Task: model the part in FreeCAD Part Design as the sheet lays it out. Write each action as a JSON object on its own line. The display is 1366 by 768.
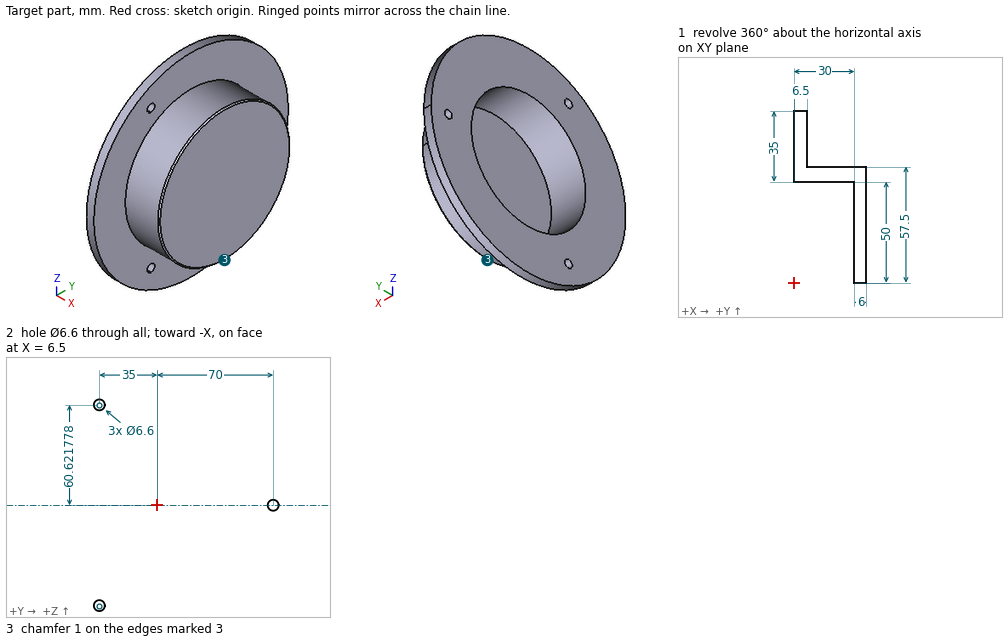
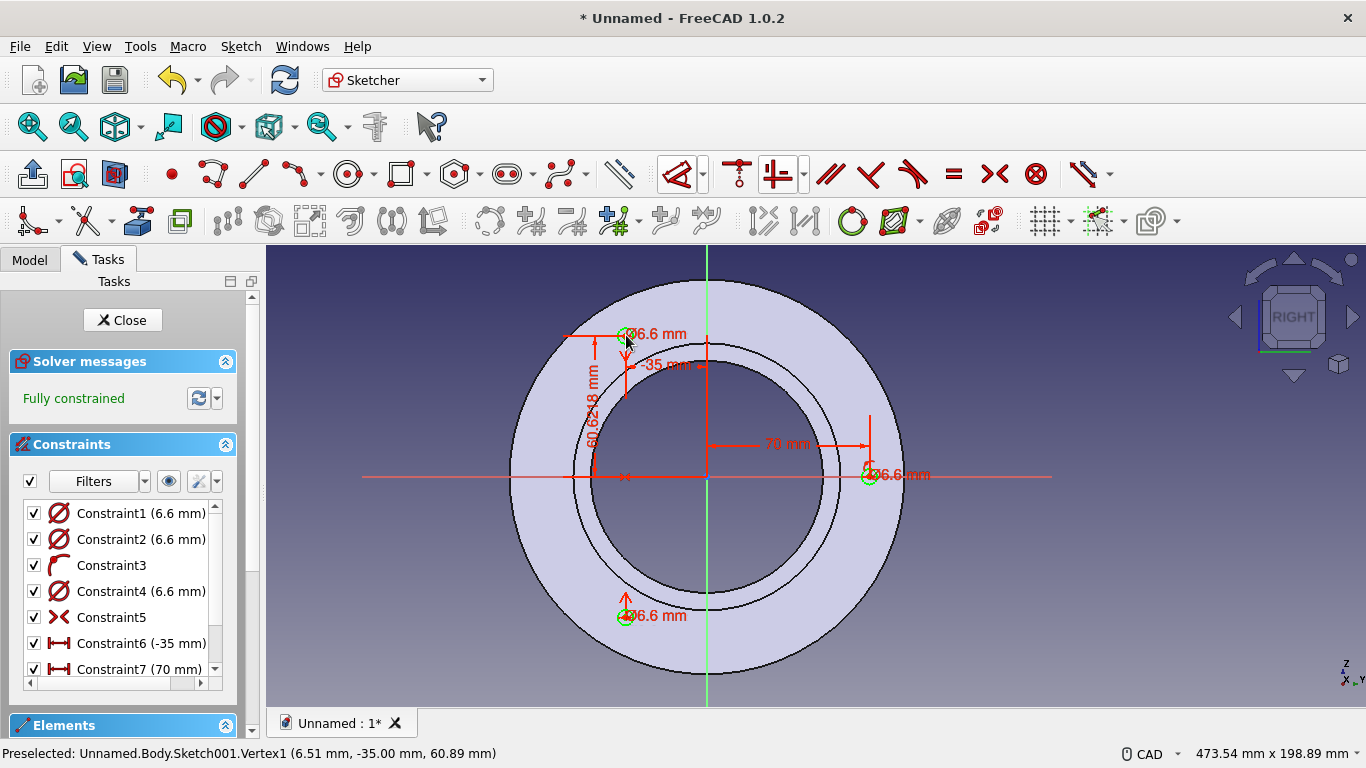
{"action": "left_click", "coordinate": [123, 320]}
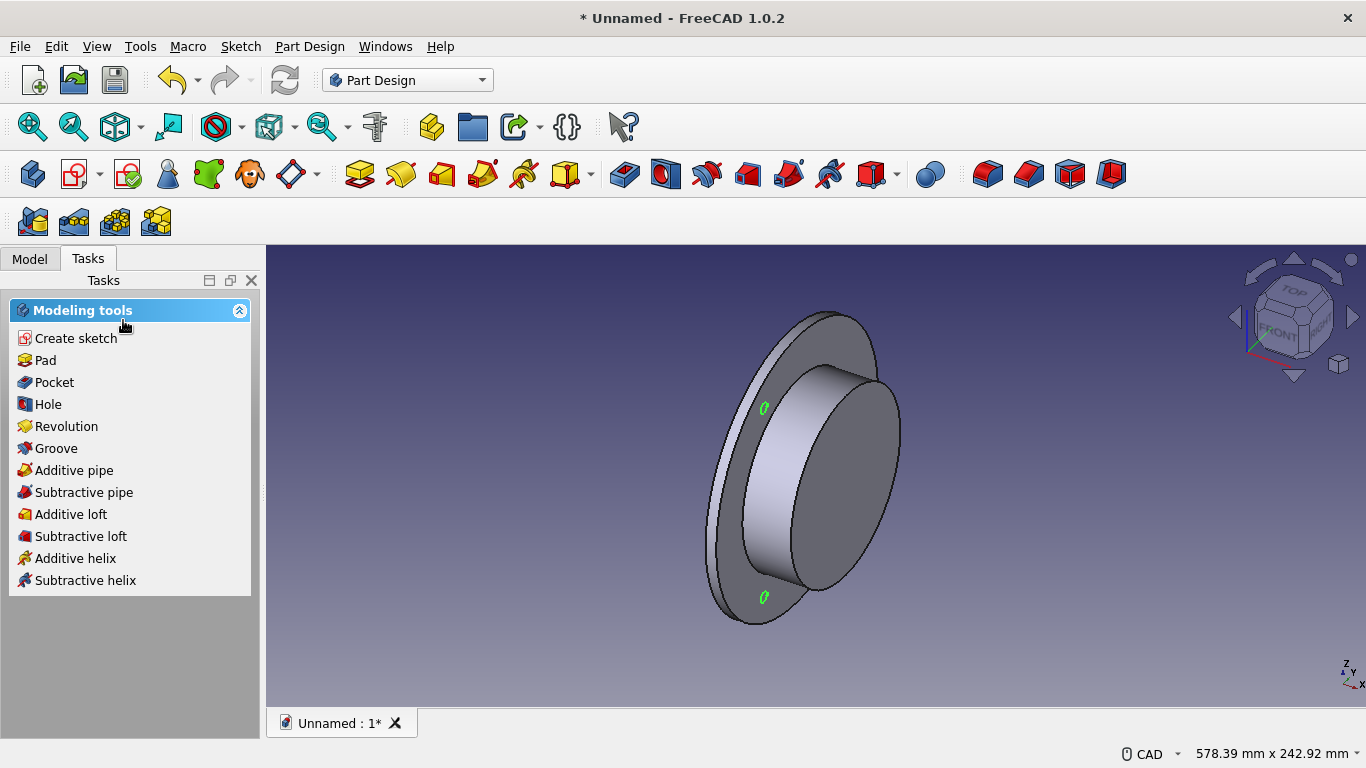
{"action": "left_click", "coordinate": [666, 174]}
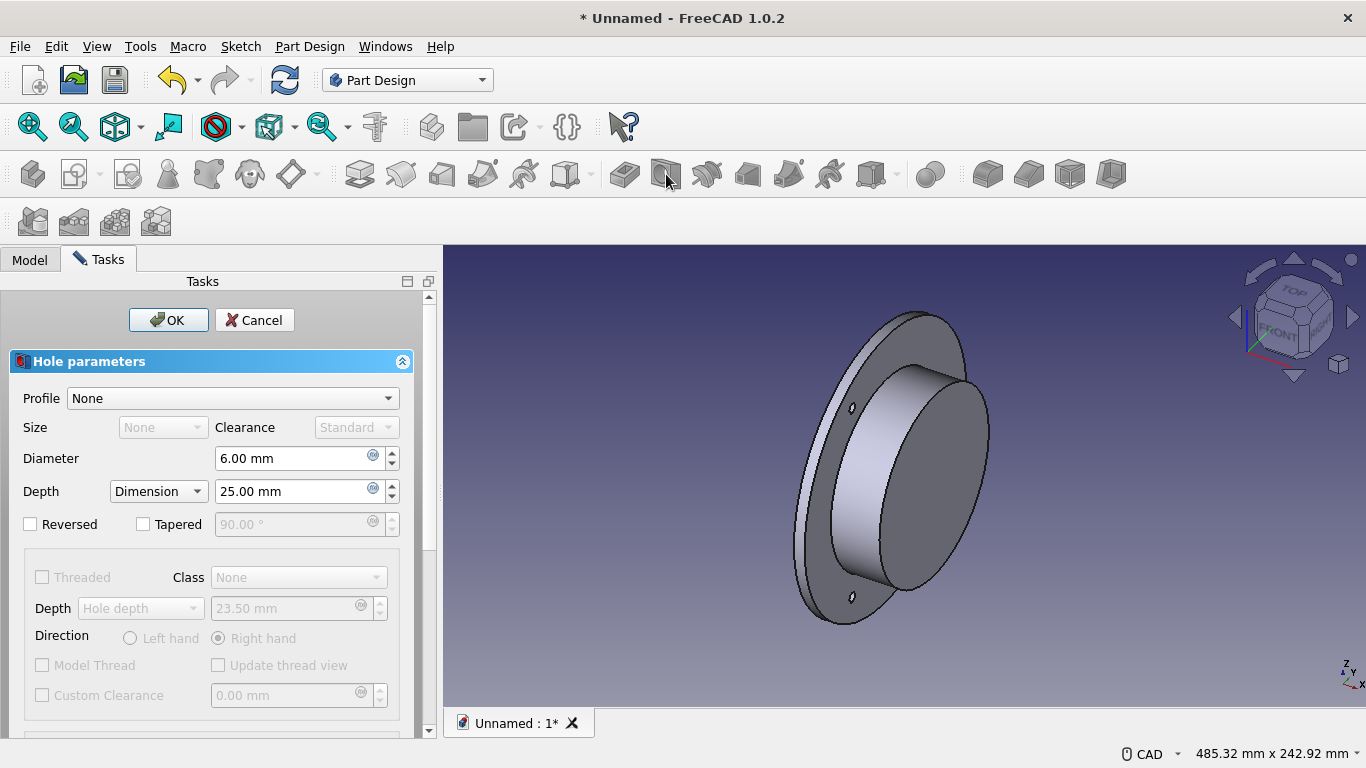
{"action": "triple_click", "coordinate": [300, 458]}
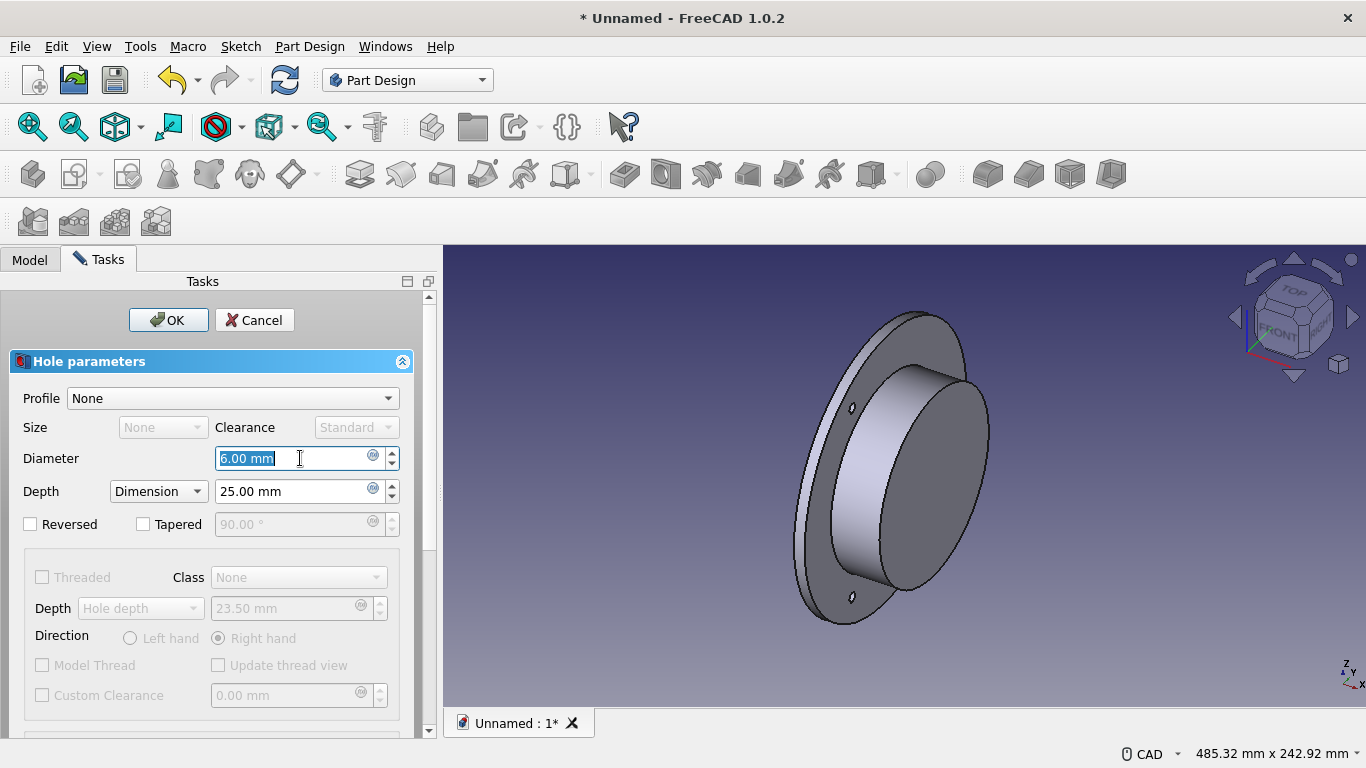
{"action": "type", "text": "6.6"}
{"action": "key", "text": "Tab"}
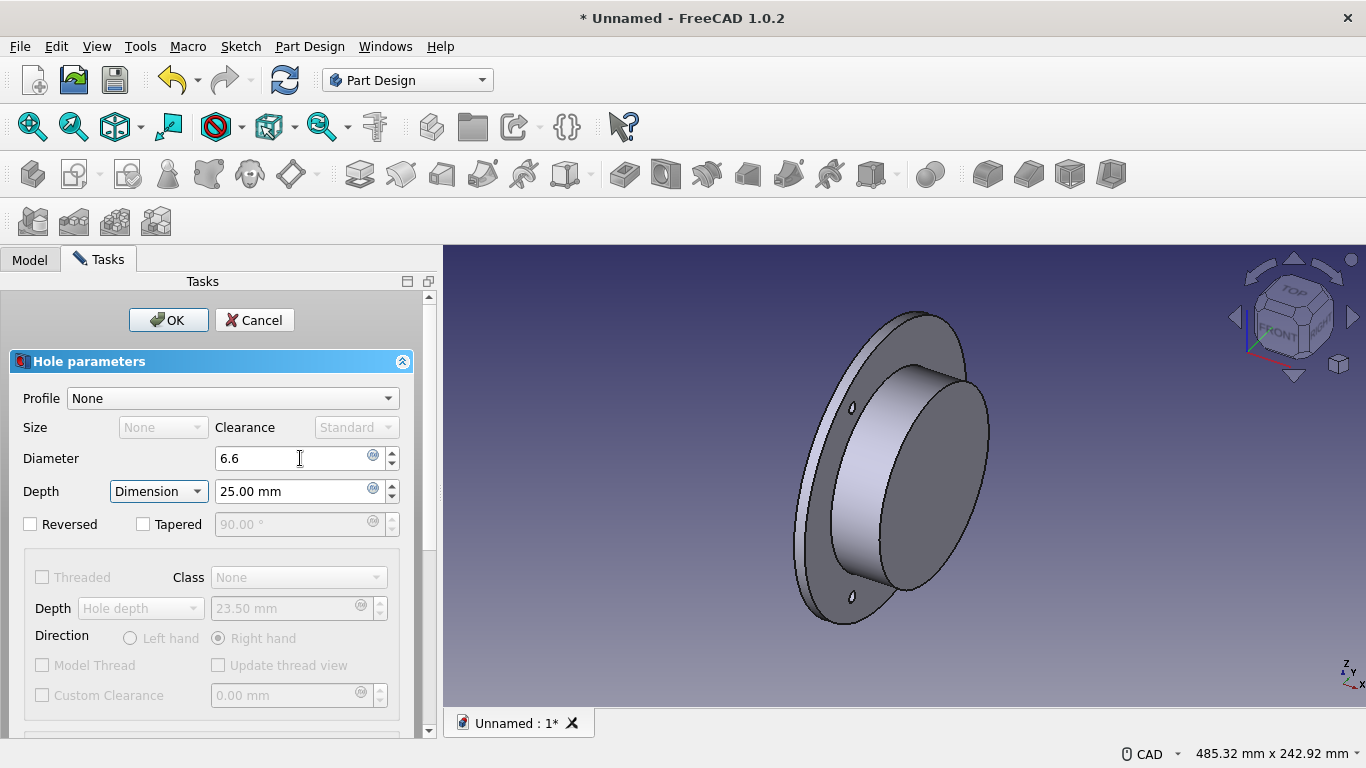
{"action": "left_click", "coordinate": [160, 492]}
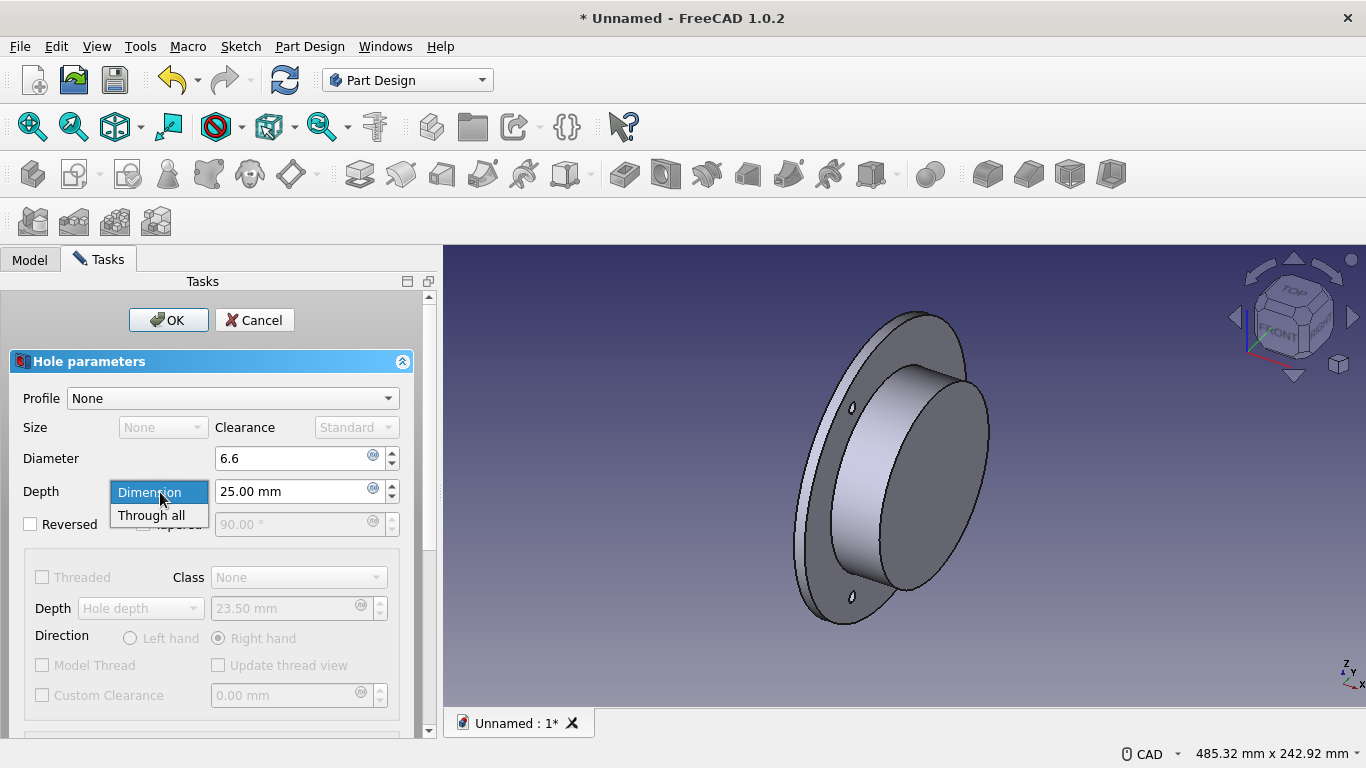
{"action": "left_click", "coordinate": [158, 516]}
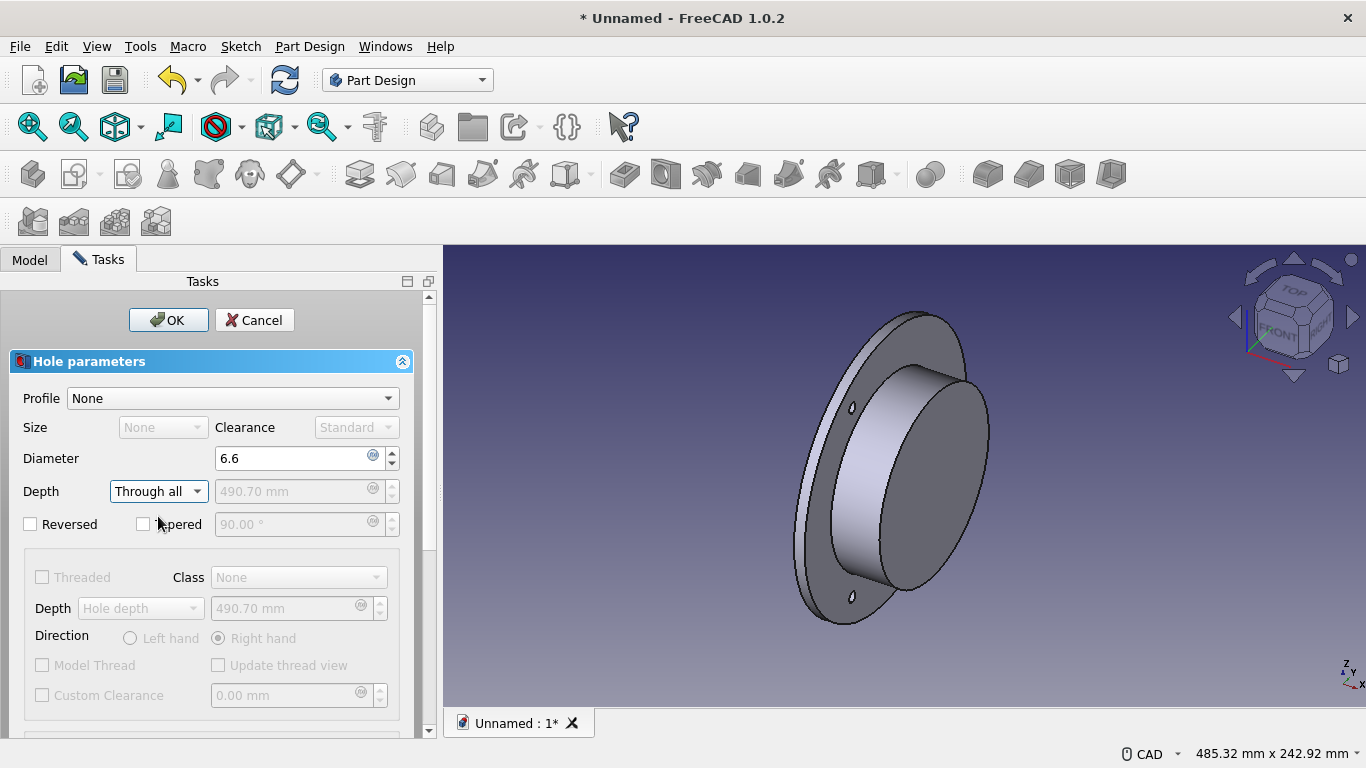
{"action": "left_click", "coordinate": [169, 320]}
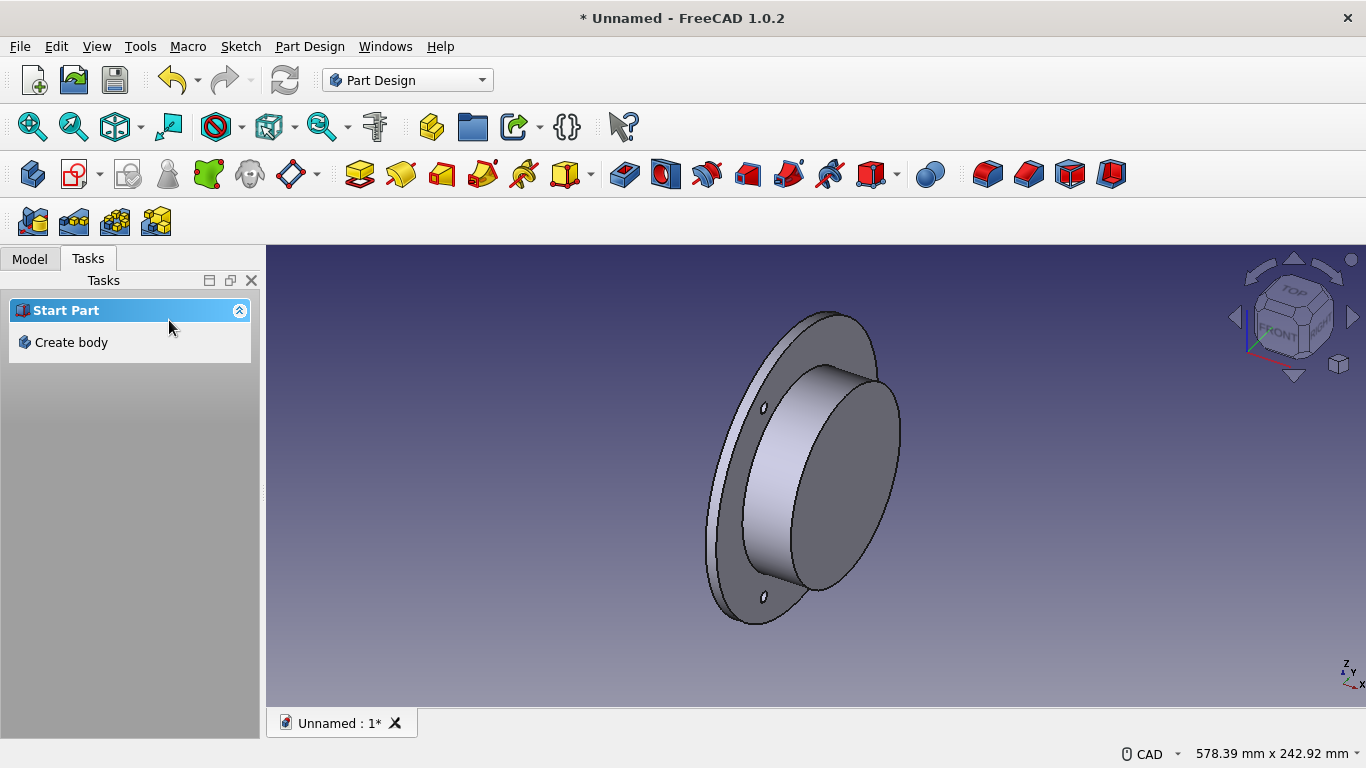
{"action": "left_click", "coordinate": [791, 539]}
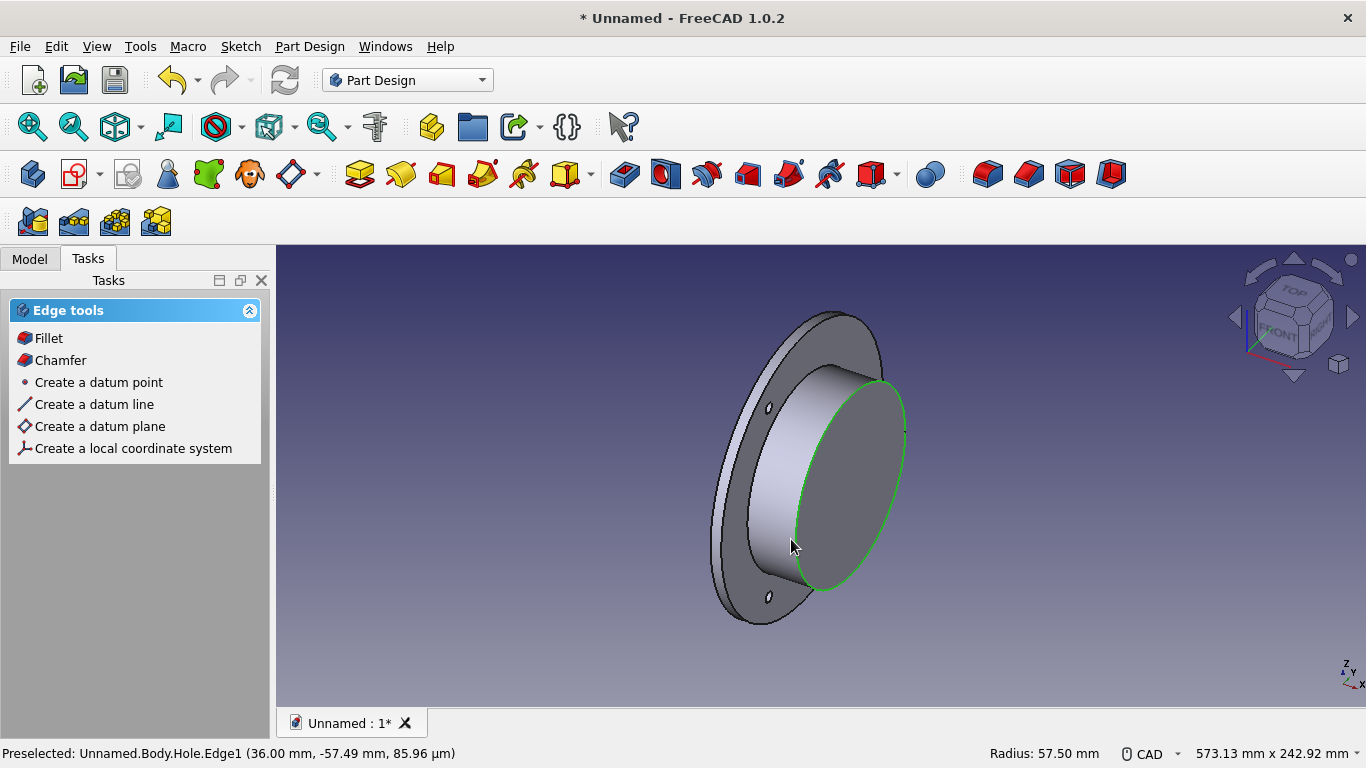
{"action": "left_click", "coordinate": [1029, 174]}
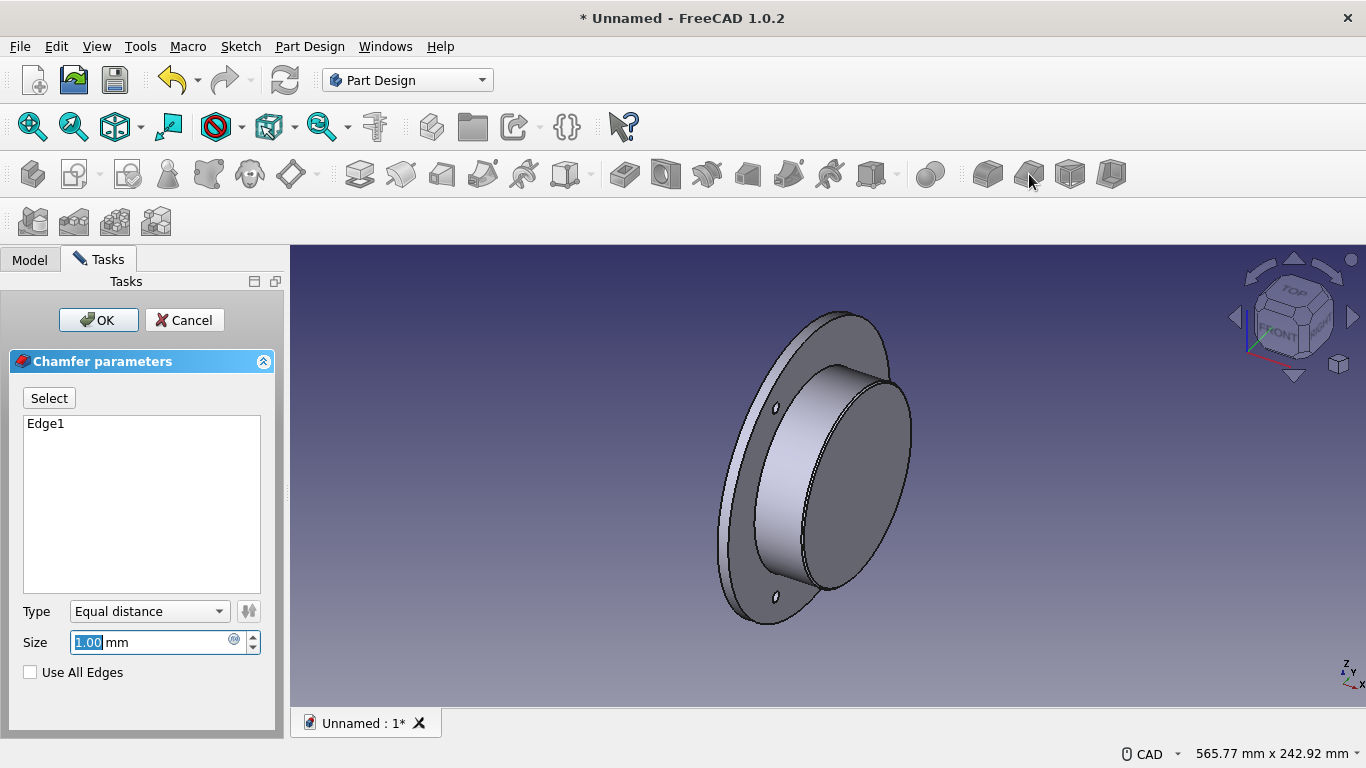
{"action": "type", "text": "1"}
{"action": "key", "text": "Tab"}